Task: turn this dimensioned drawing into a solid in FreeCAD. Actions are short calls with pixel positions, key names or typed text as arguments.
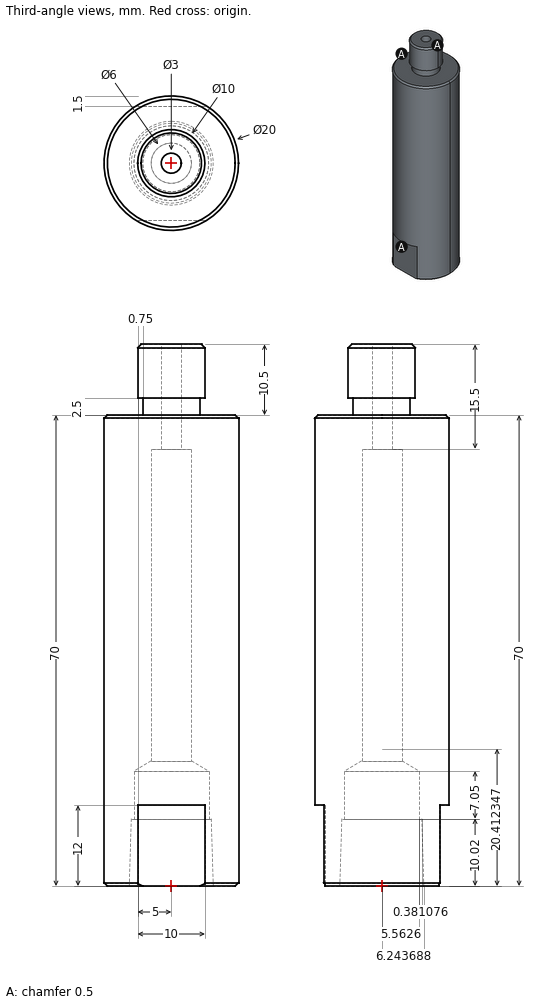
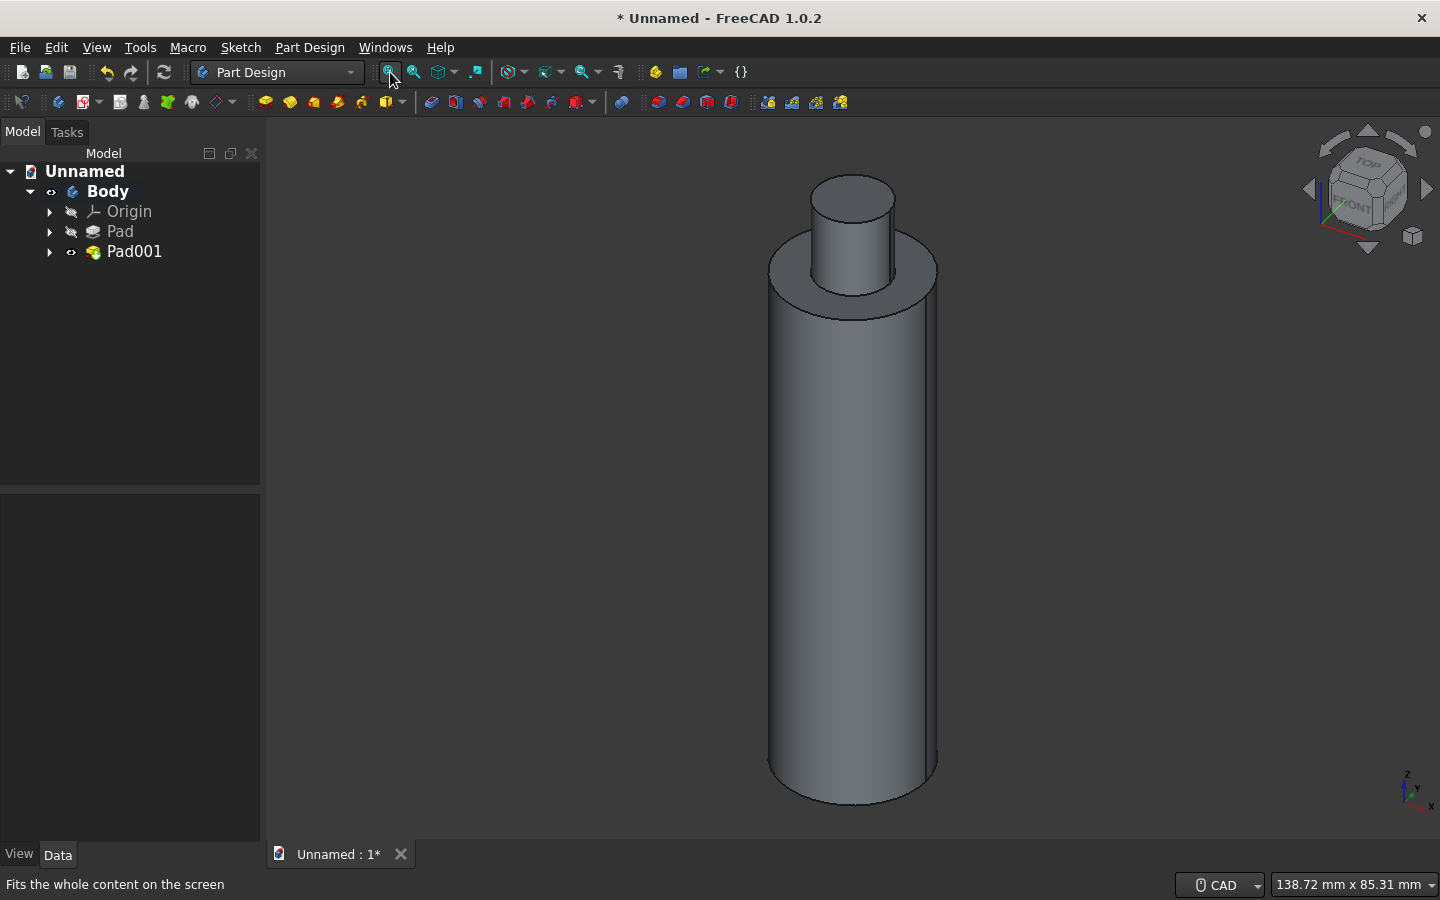
click(84, 102)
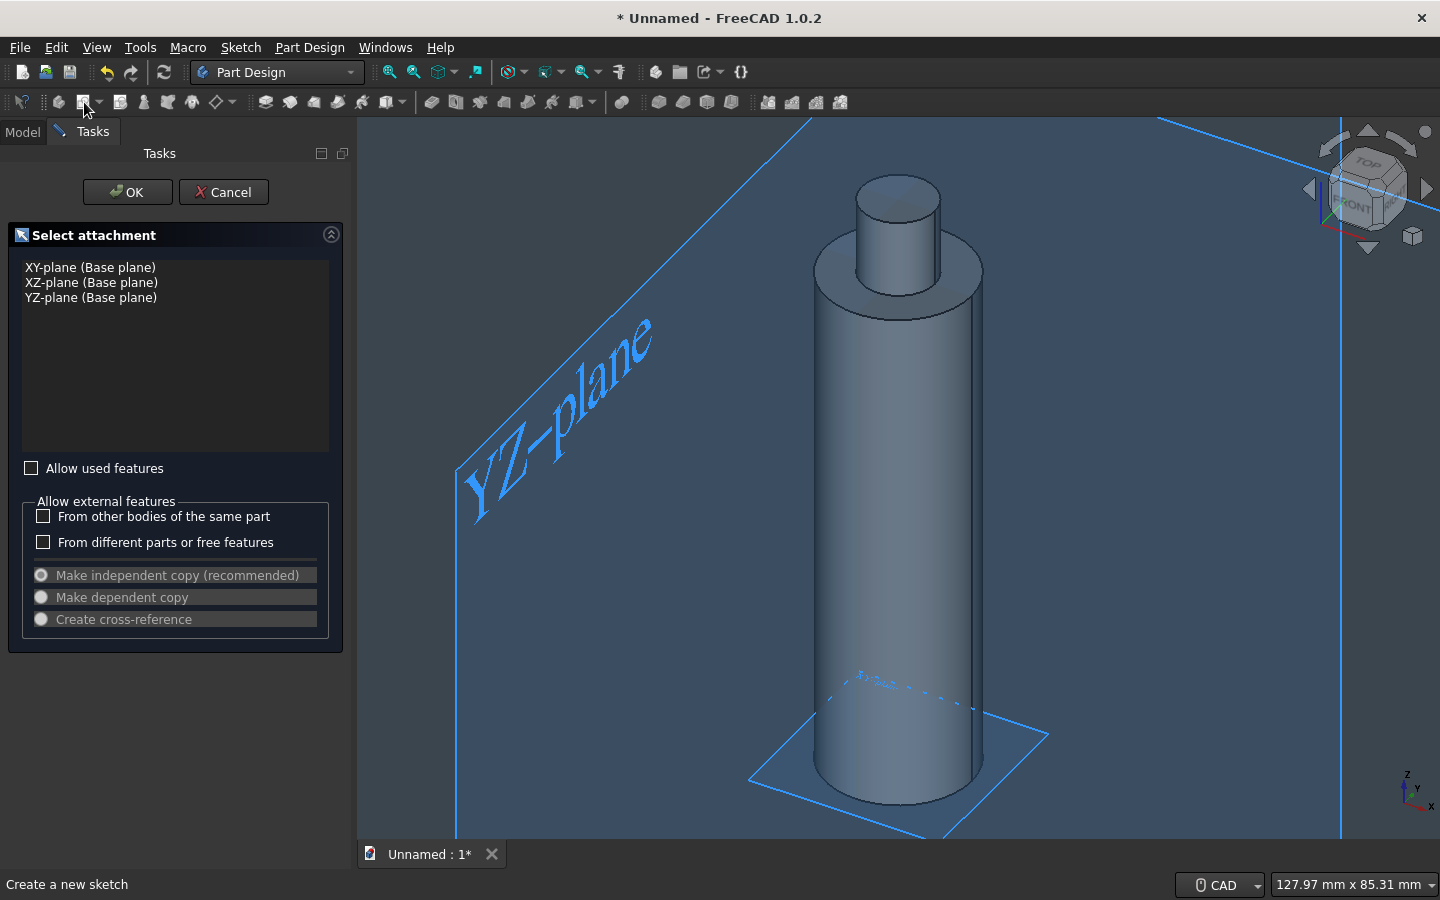
click(82, 282)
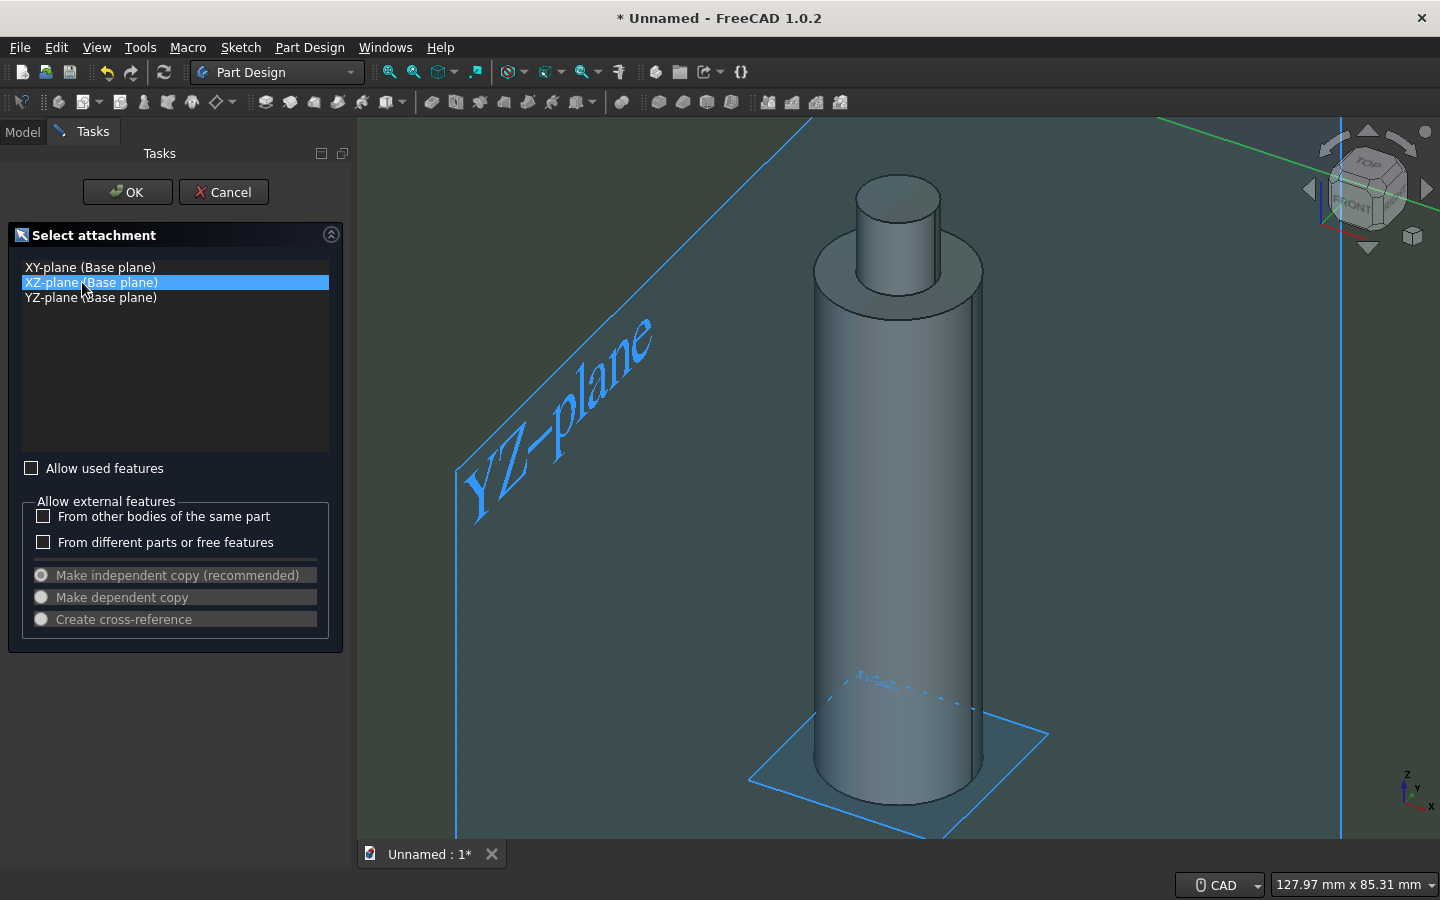
click(128, 192)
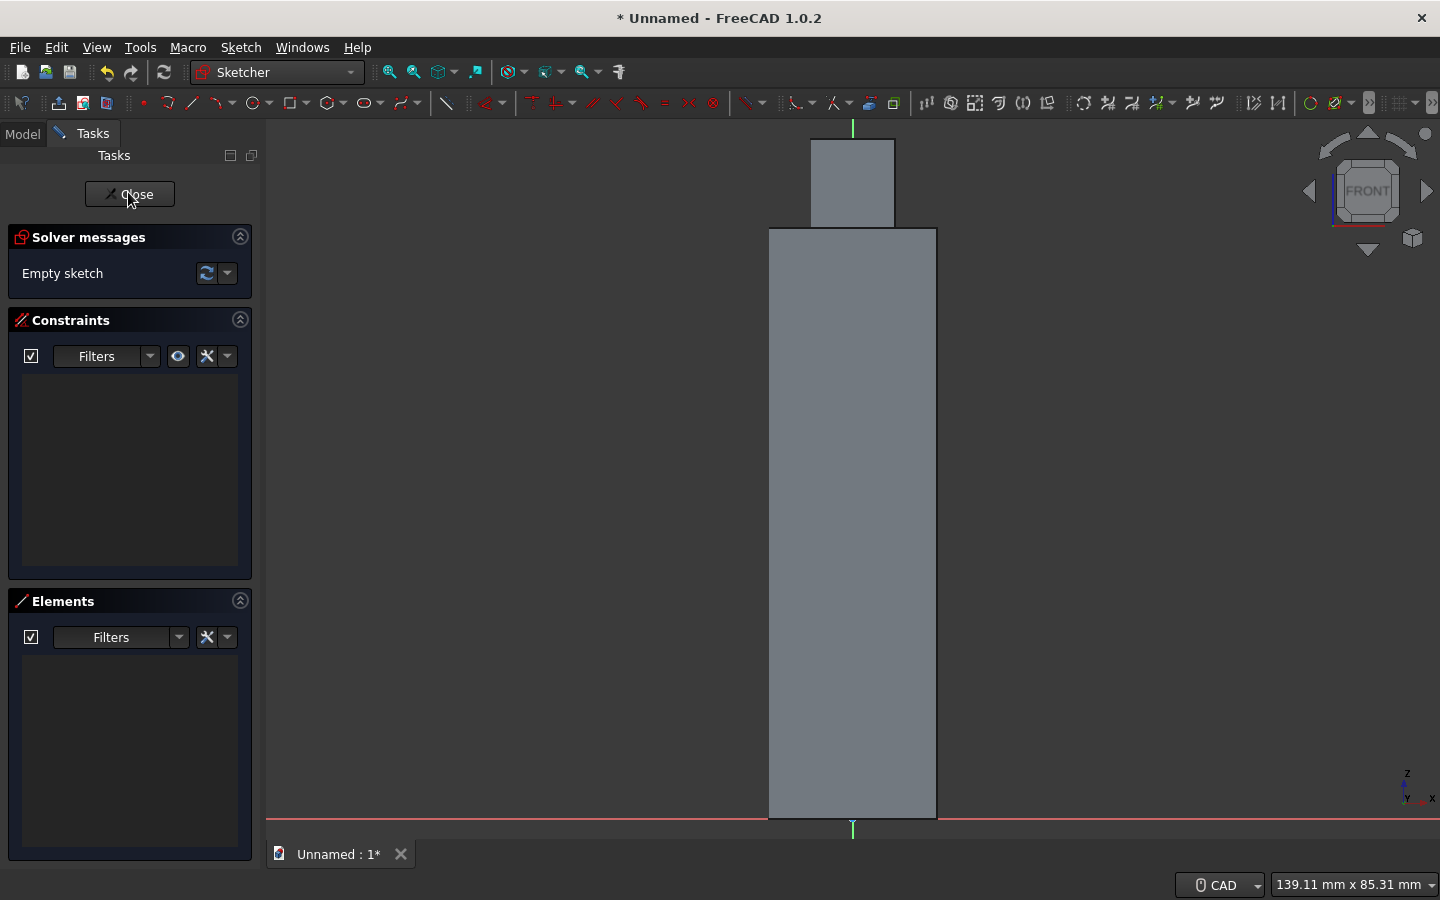
click(108, 104)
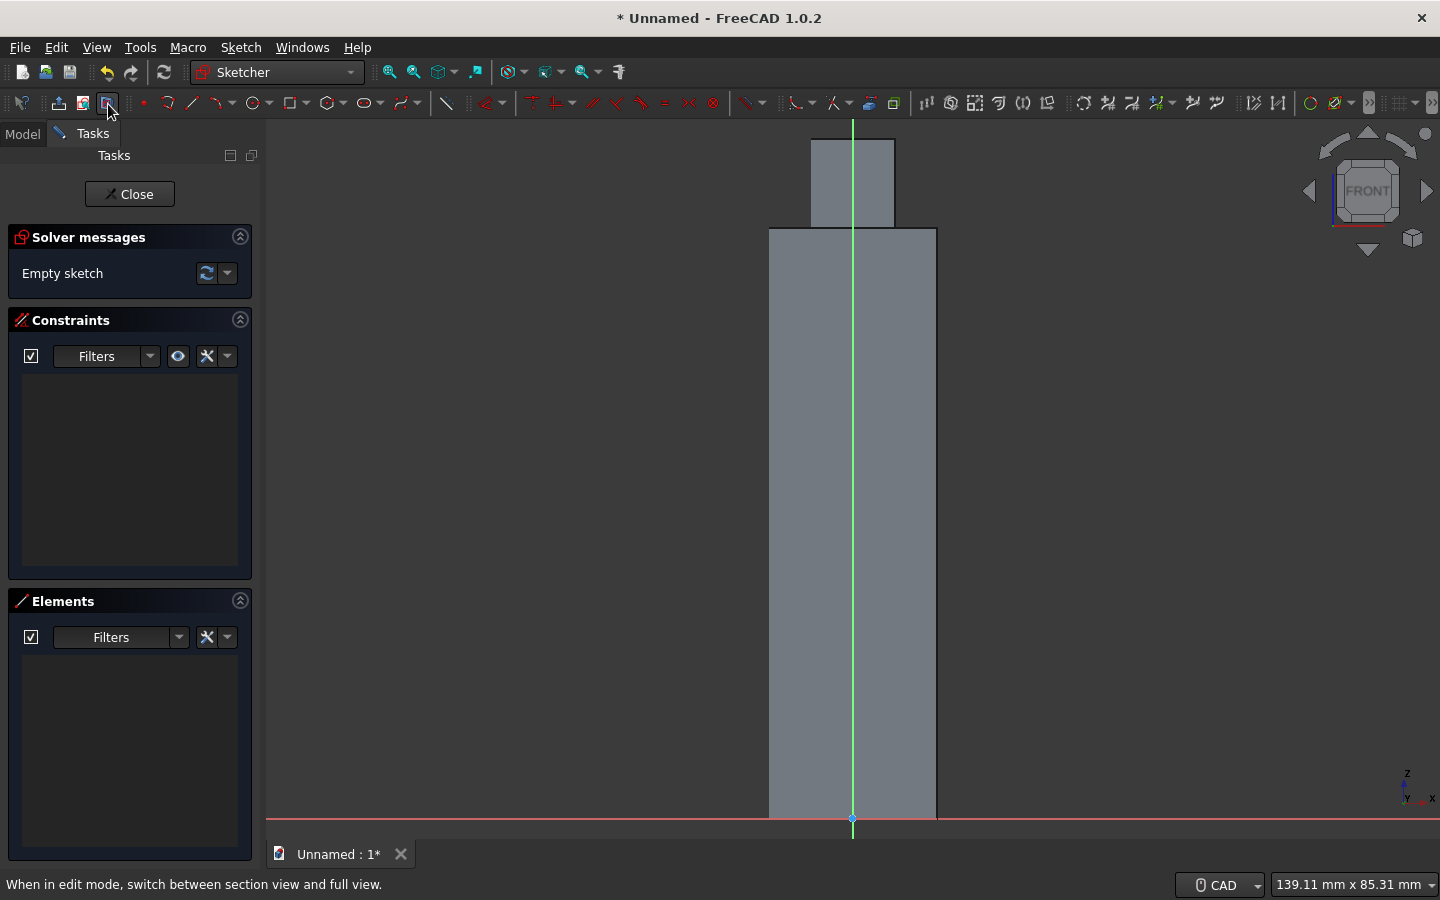
scroll(815, 204, up, 15)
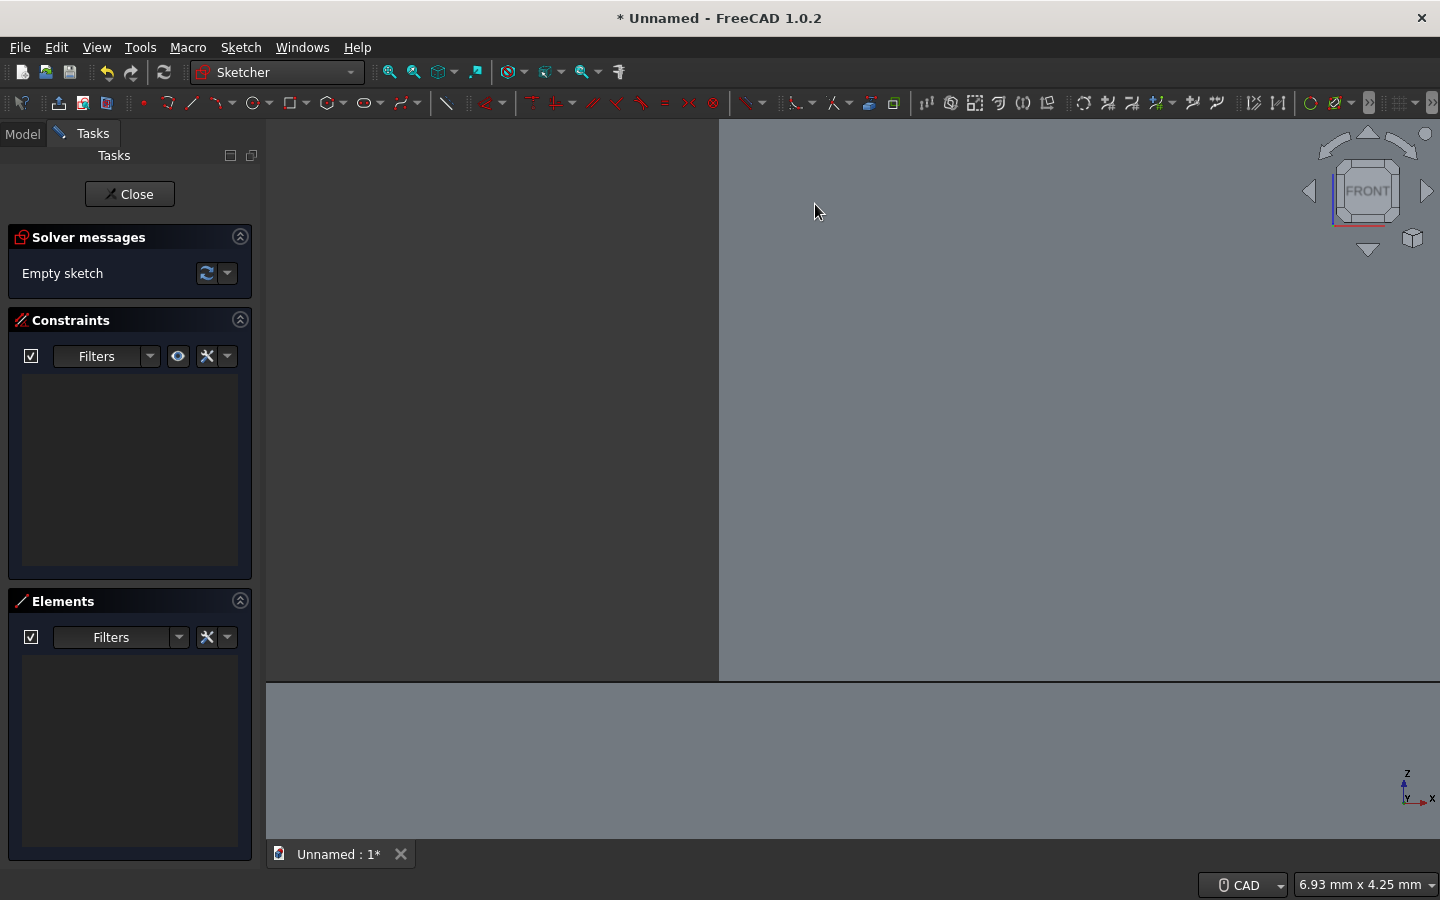
click(290, 104)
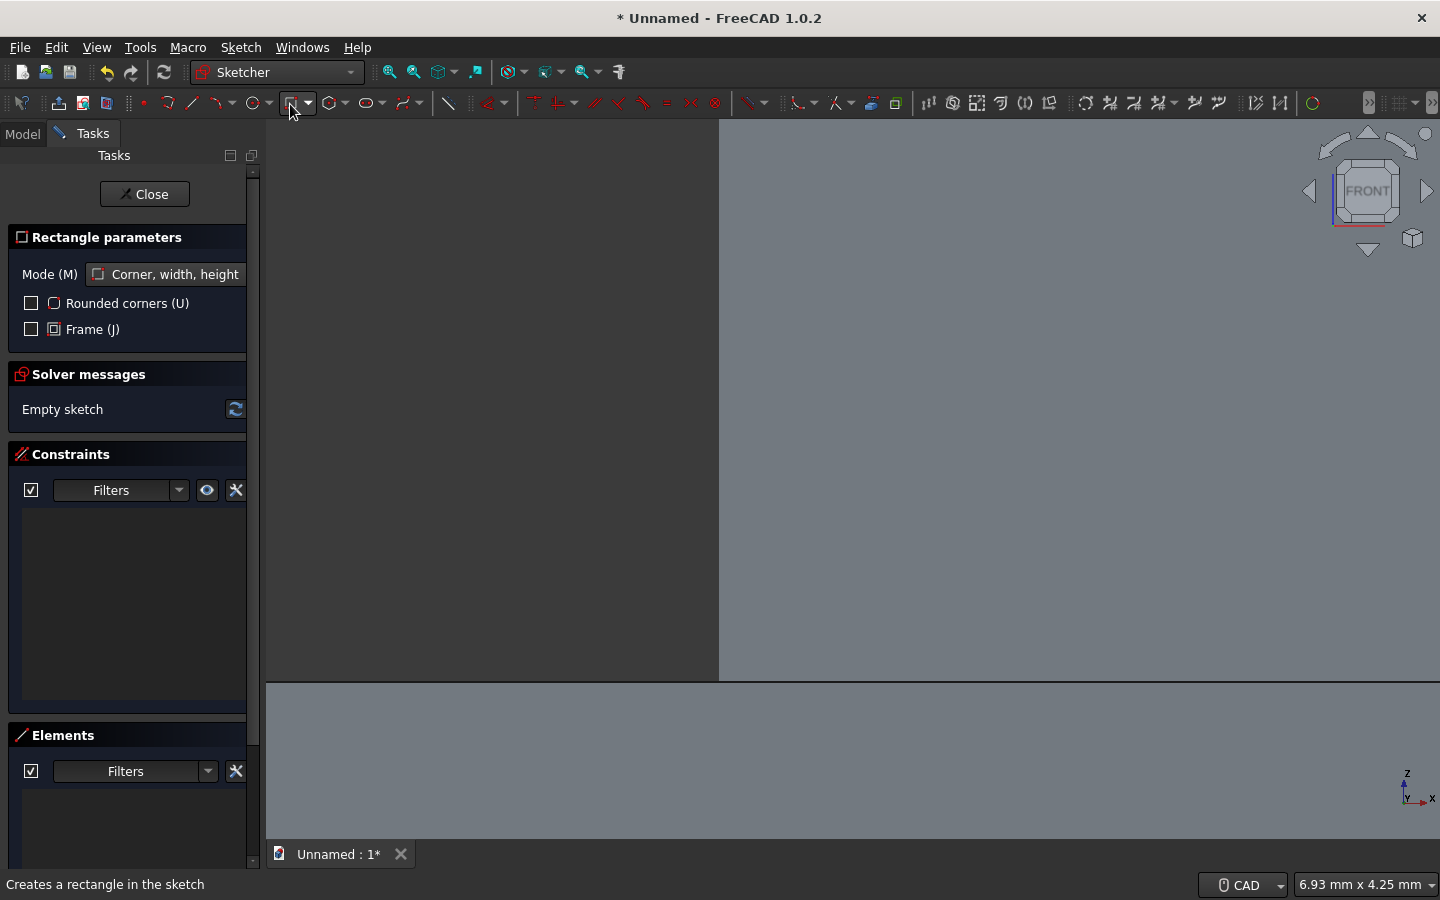
click(719, 258)
move(846, 682)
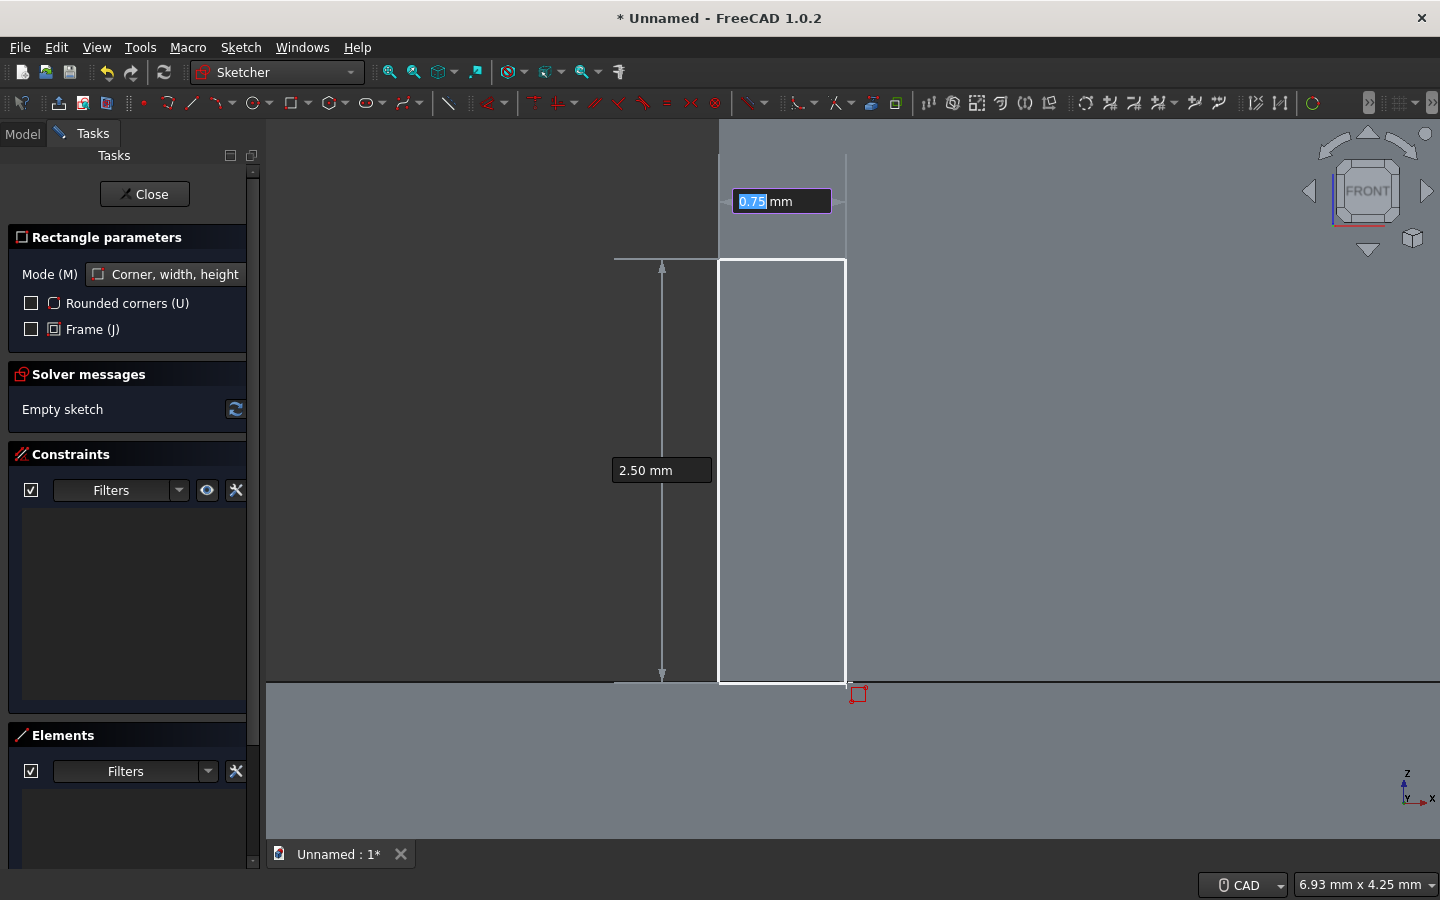
text(0.75)
key(Tab)
text(2.5)
key(Return)
key(Escape)